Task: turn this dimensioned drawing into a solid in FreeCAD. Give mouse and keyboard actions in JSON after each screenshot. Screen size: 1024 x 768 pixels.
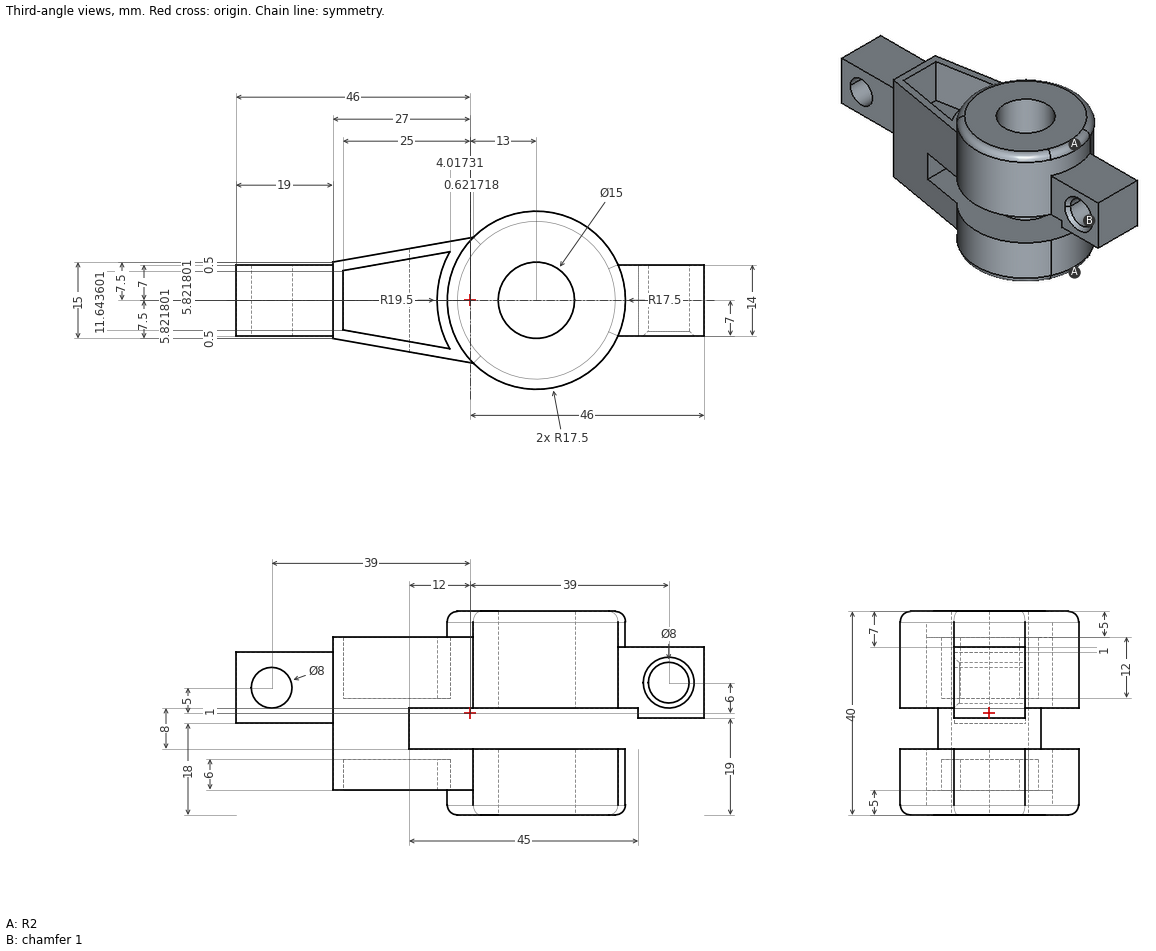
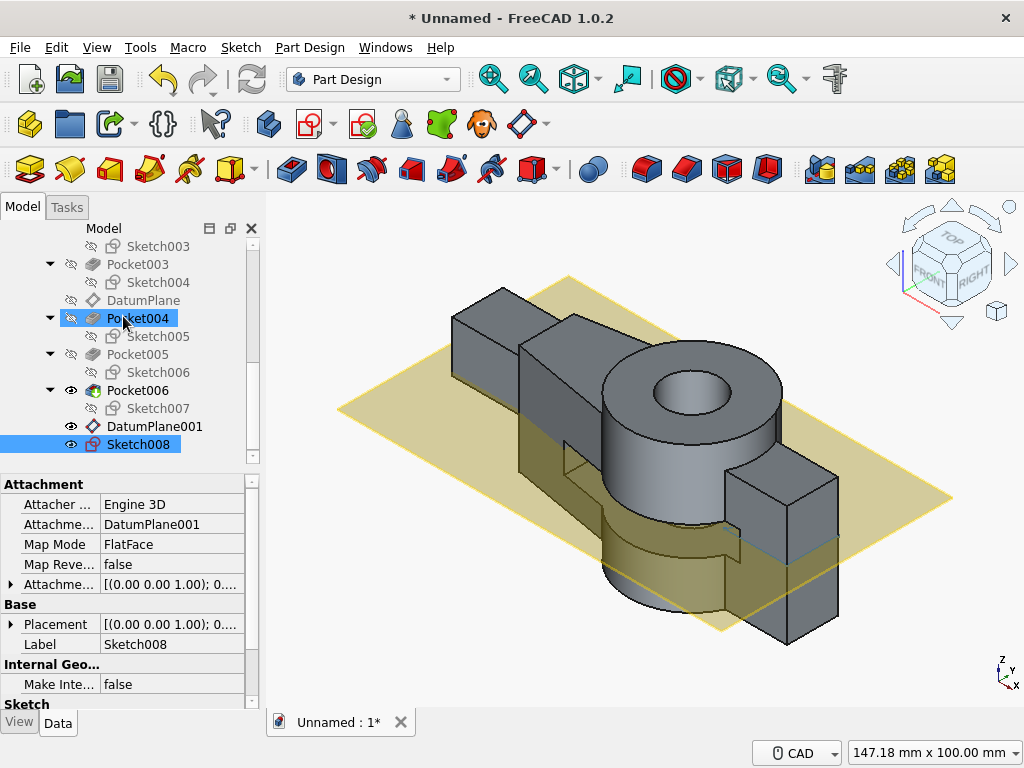
{"action": "left_click", "coordinate": [292, 170]}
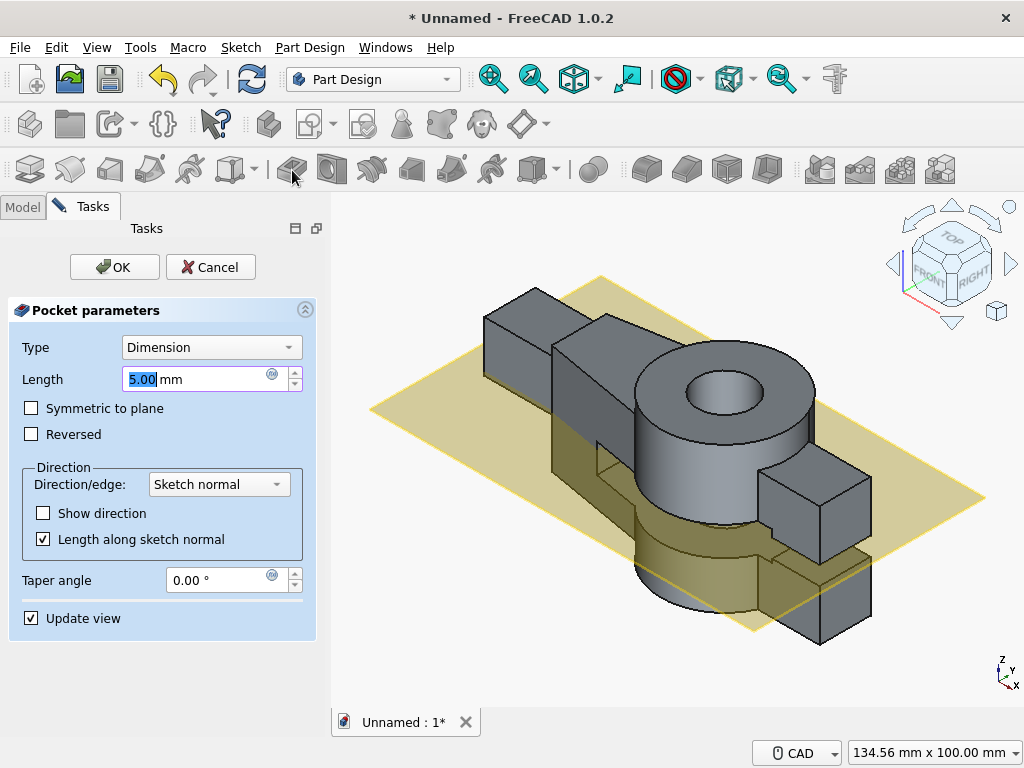
{"action": "type", "text": "19"}
{"action": "key", "text": "Tab"}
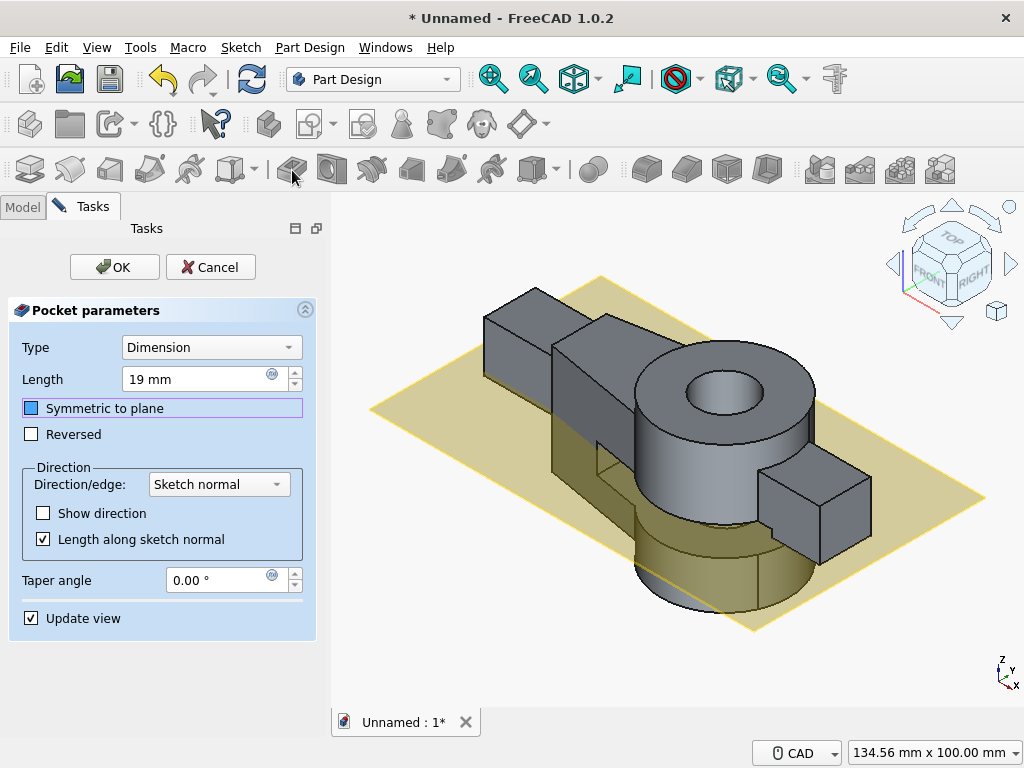
{"action": "left_click", "coordinate": [115, 267]}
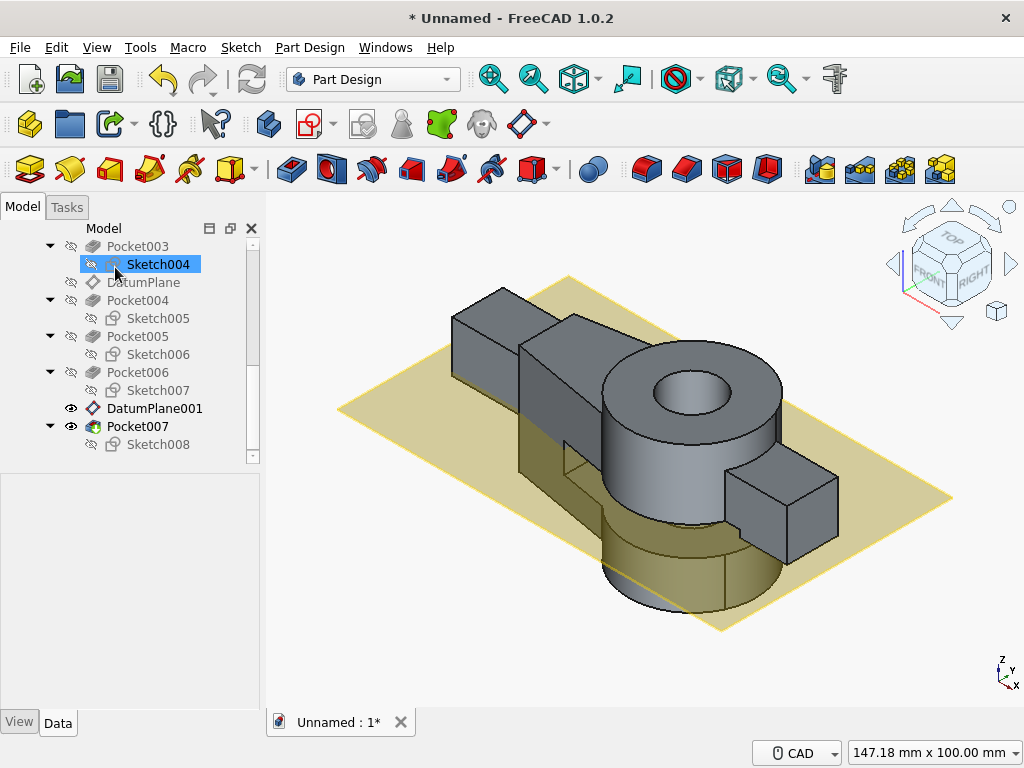
{"action": "left_click", "coordinate": [116, 408]}
{"action": "key", "text": "space"}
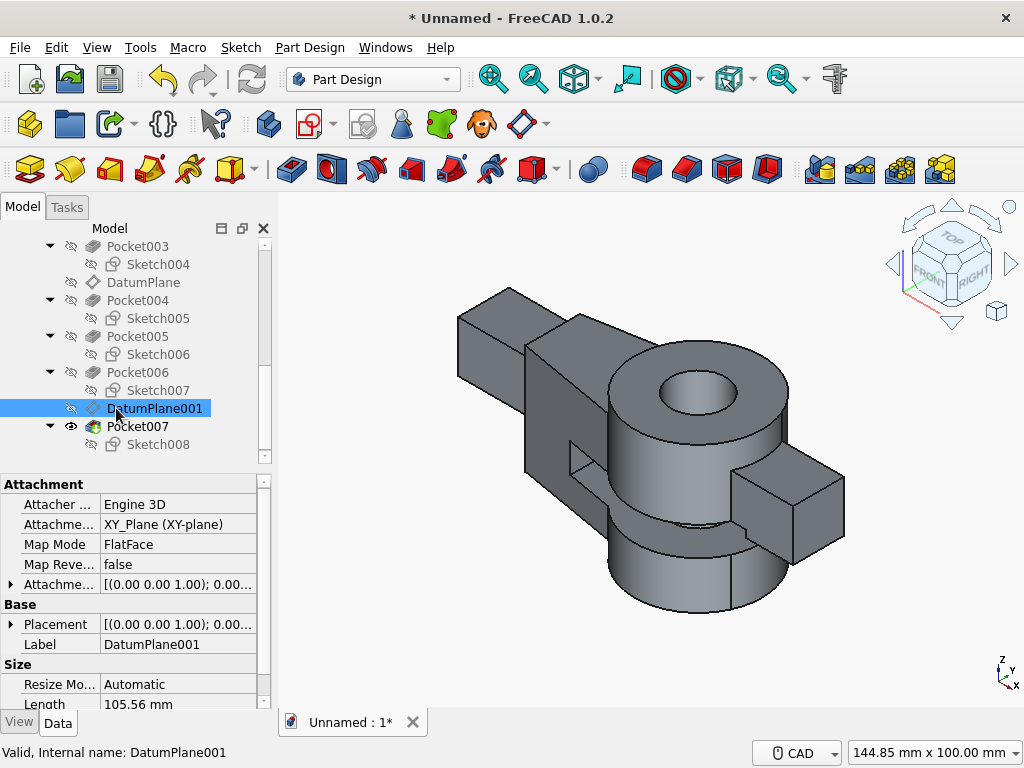
{"action": "left_click", "coordinate": [589, 349]}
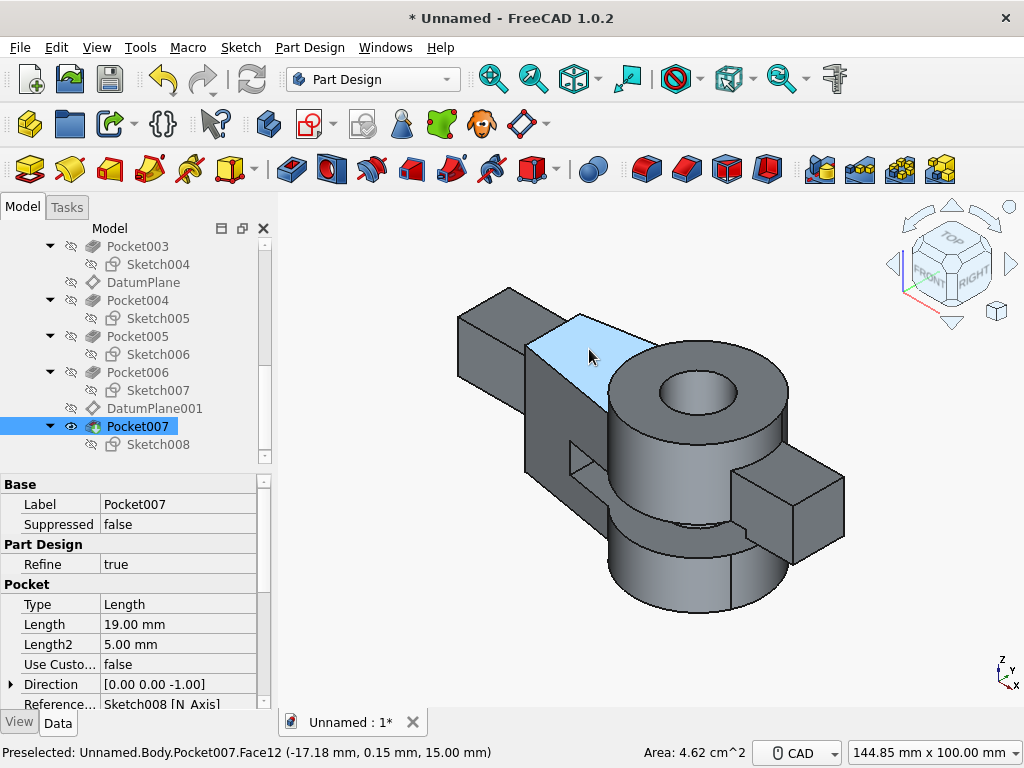
{"action": "left_click", "coordinate": [310, 124]}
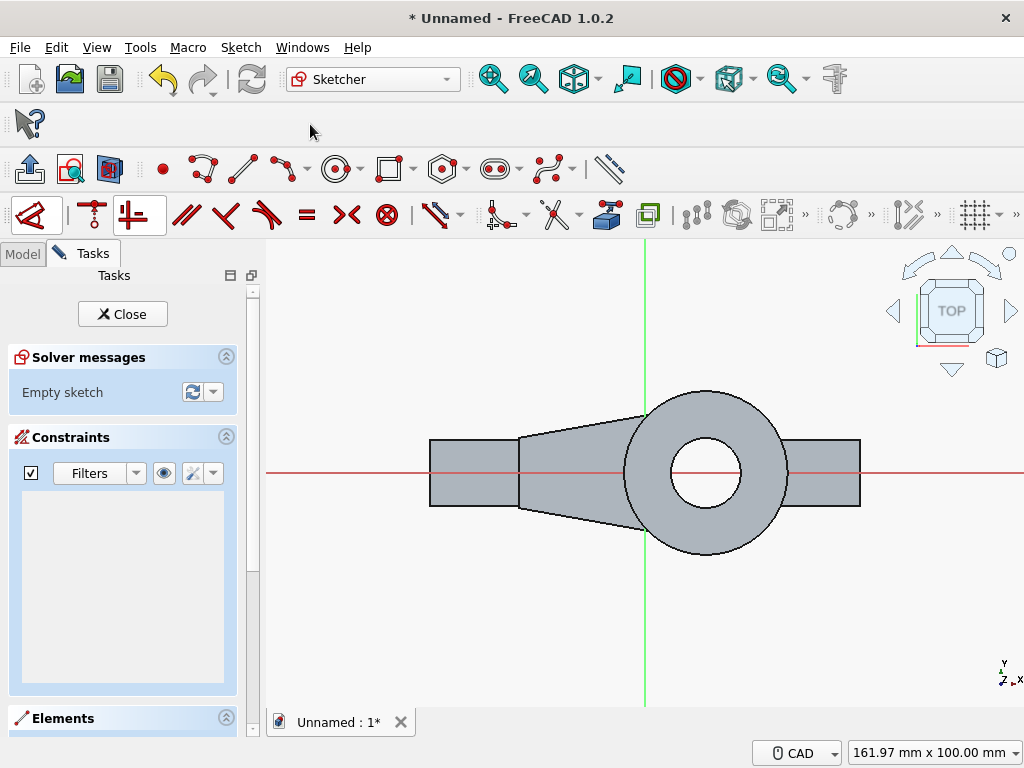
{"action": "scroll", "coordinate": [591, 473], "scroll_direction": "up", "scroll_amount": 6}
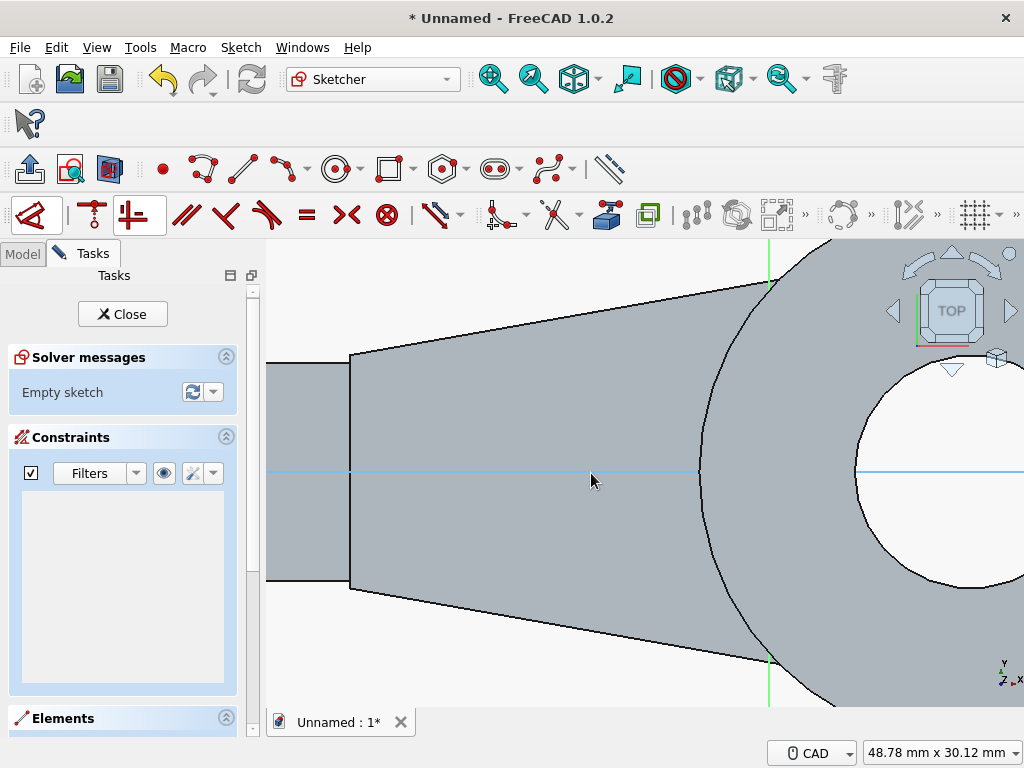
{"action": "left_click", "coordinate": [204, 170]}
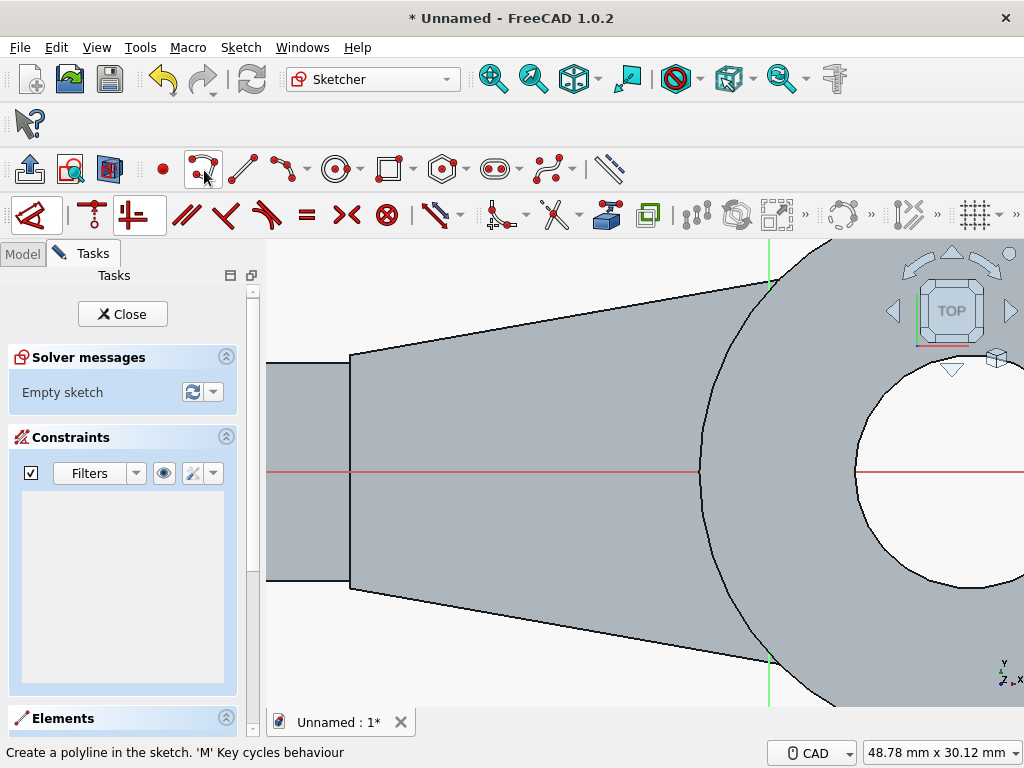
{"action": "left_click", "coordinate": [707, 324]}
{"action": "left_click", "coordinate": [381, 381]}
{"action": "left_click", "coordinate": [381, 562]}
{"action": "left_click", "coordinate": [707, 620]}
{"action": "right_click", "coordinate": [707, 620]}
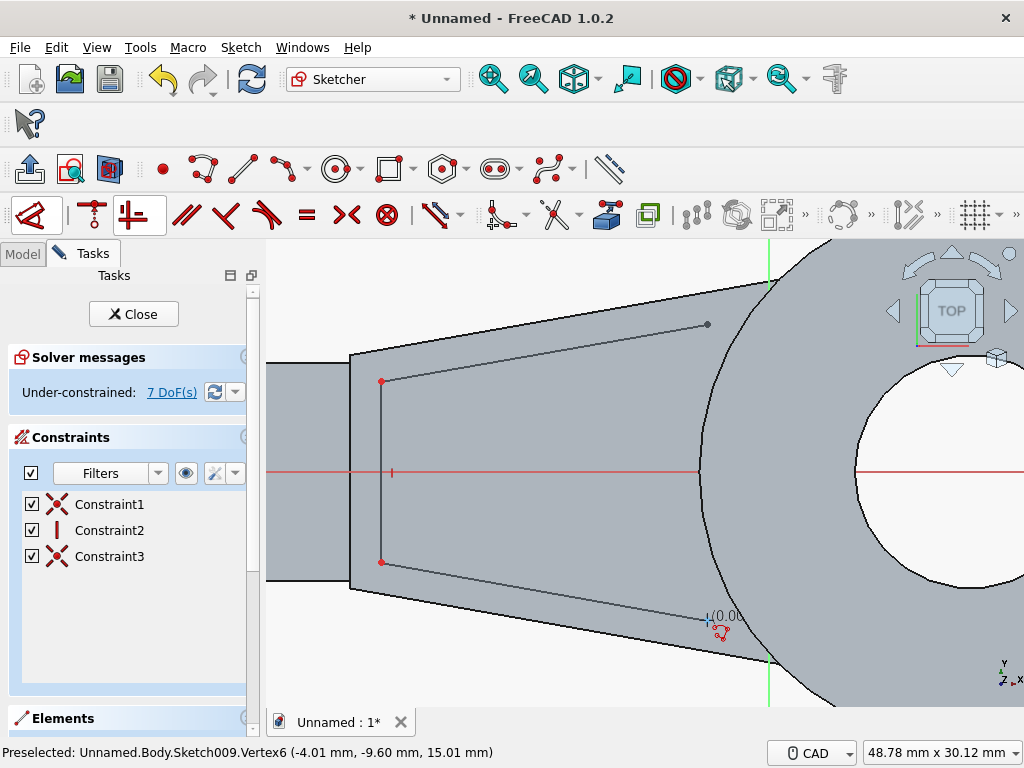
{"action": "left_click", "coordinate": [284, 170]}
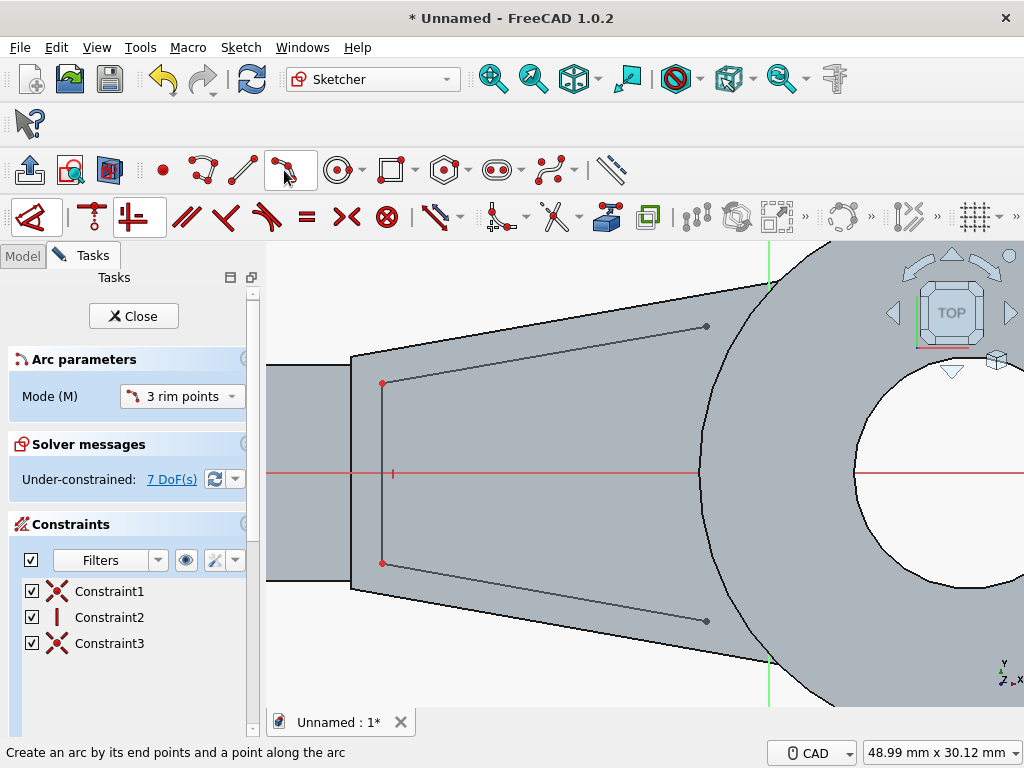
{"action": "left_click", "coordinate": [707, 621]}
{"action": "left_click", "coordinate": [707, 327]}
{"action": "left_click", "coordinate": [670, 442]}
{"action": "key", "text": "Escape"}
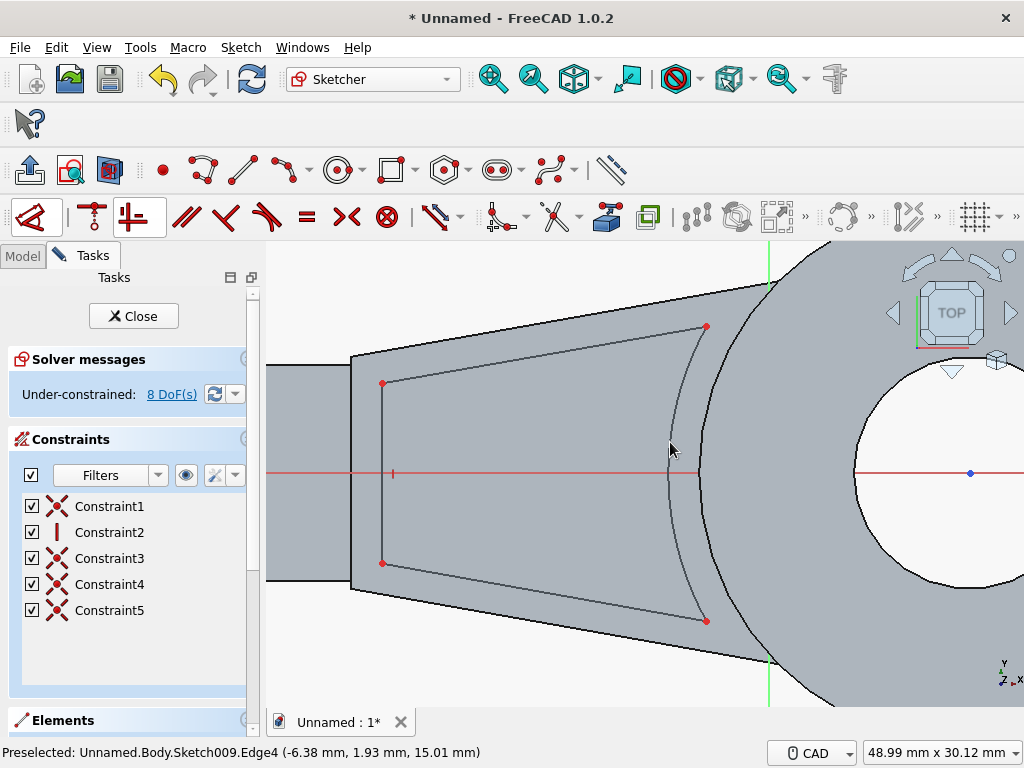
{"action": "scroll", "coordinate": [373, 476], "scroll_direction": "down", "scroll_amount": 2}